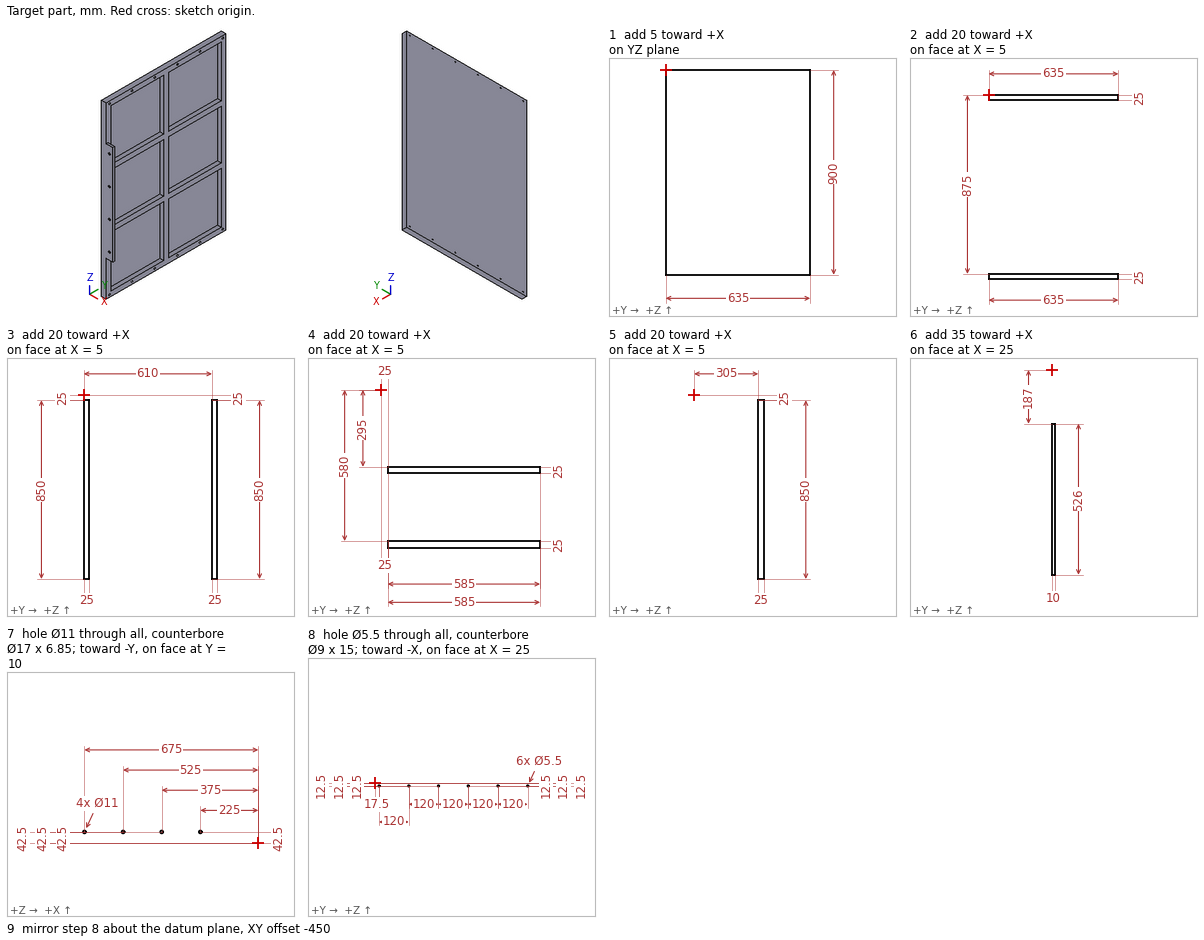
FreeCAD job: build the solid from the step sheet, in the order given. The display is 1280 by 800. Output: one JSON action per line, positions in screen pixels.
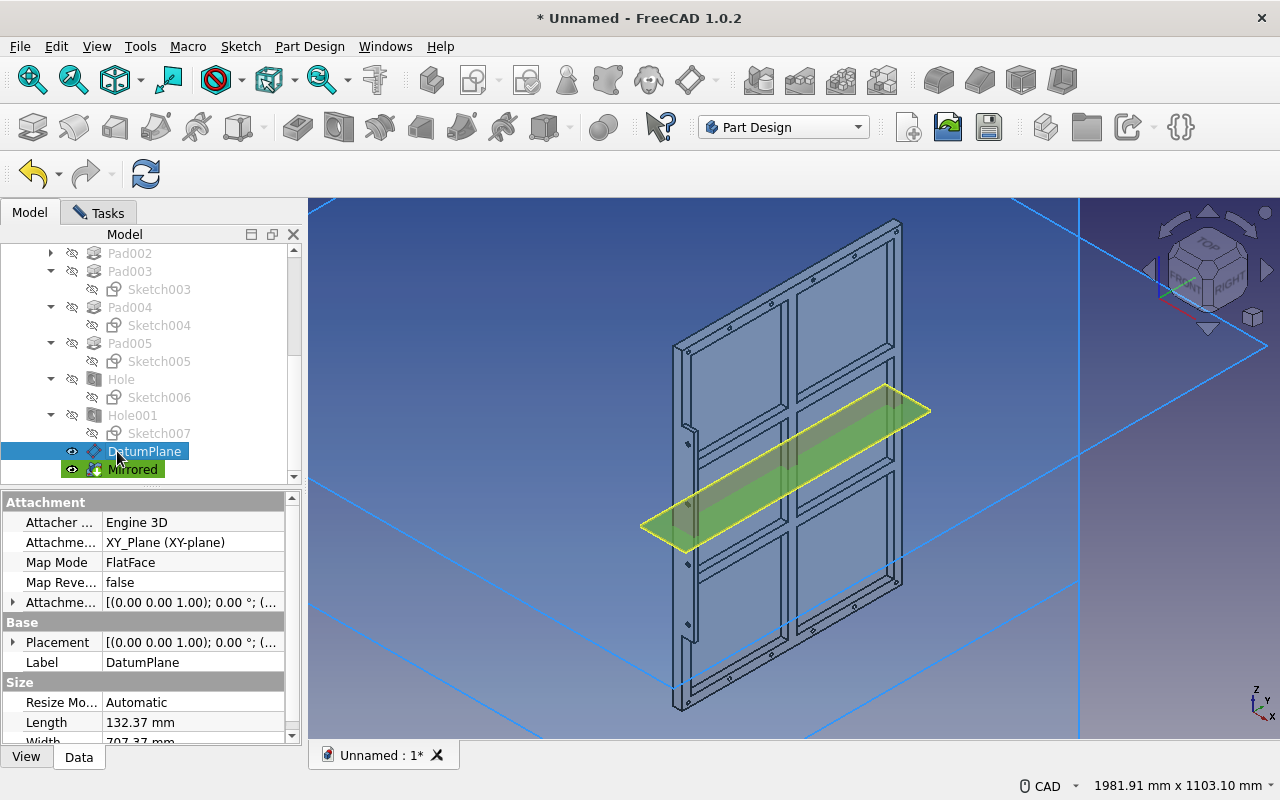
{"action": "left_click", "coordinate": [98, 212]}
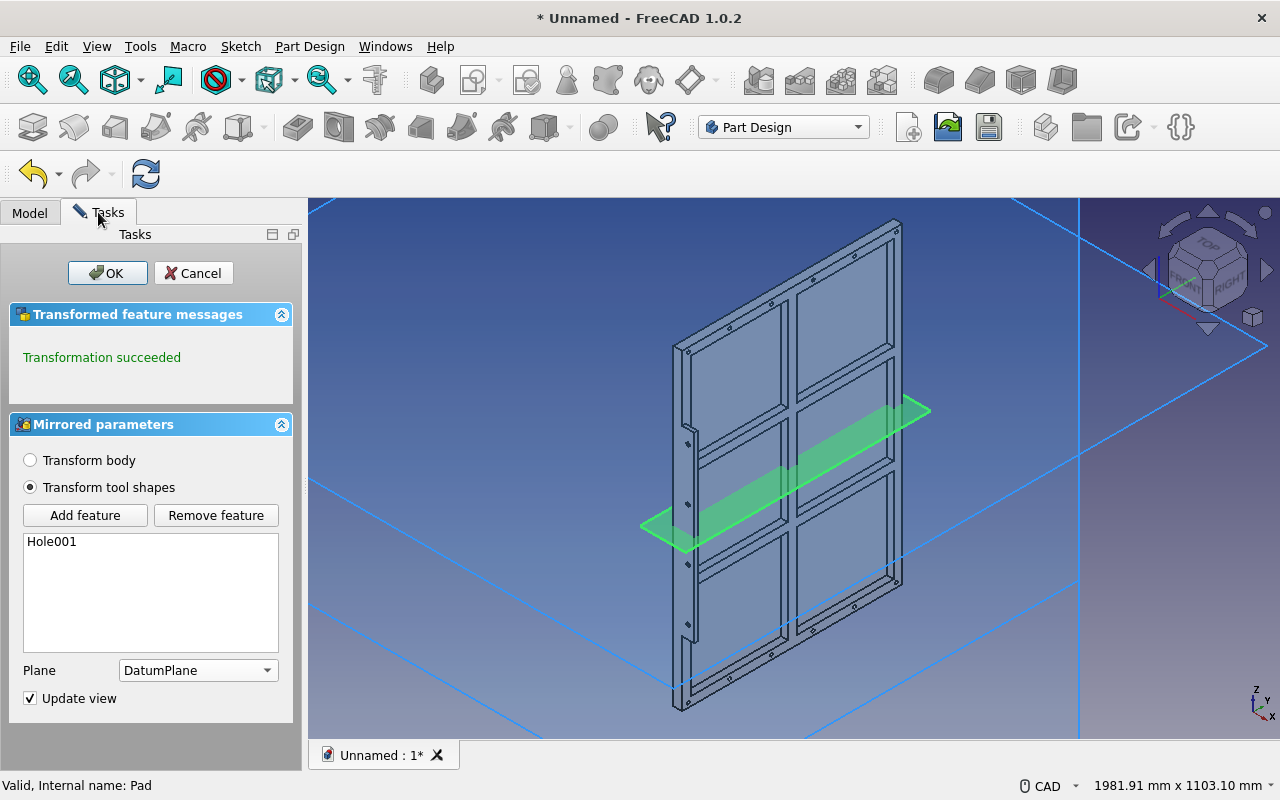
{"action": "left_click", "coordinate": [108, 273]}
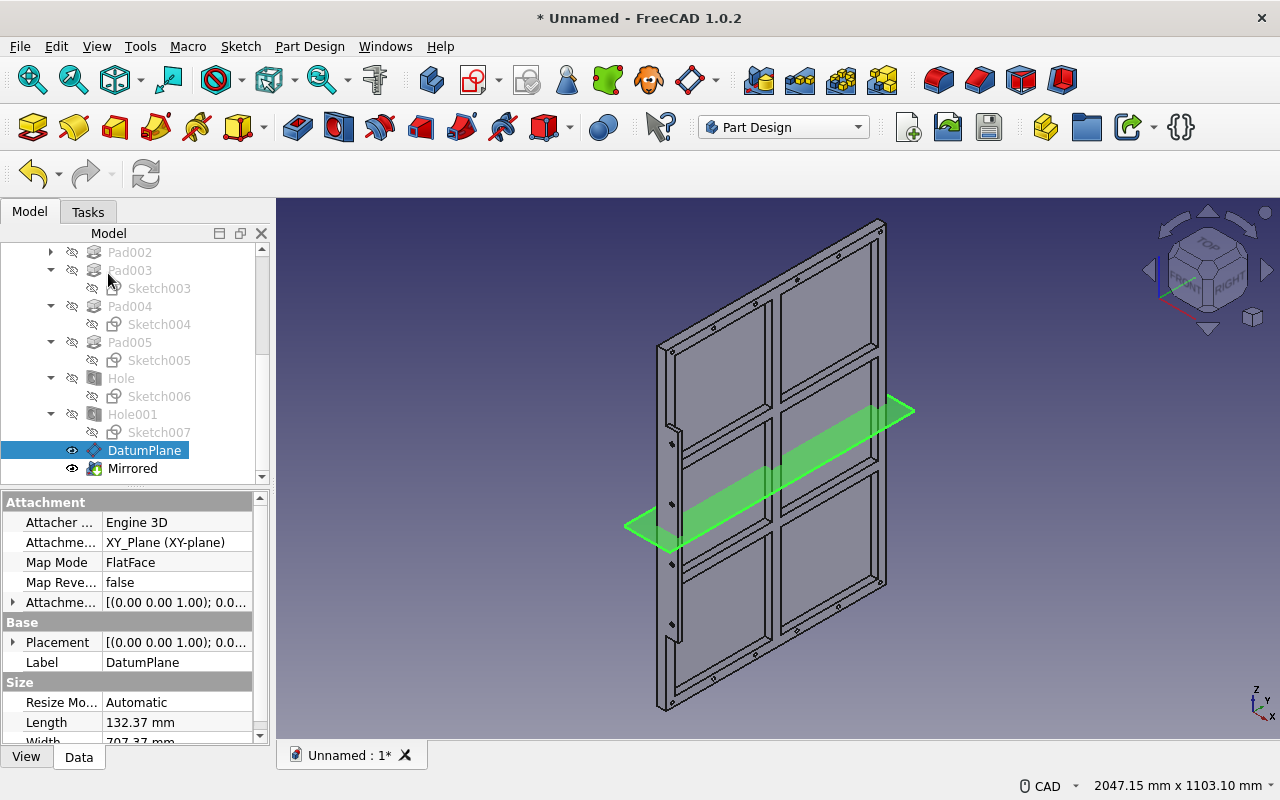
{"action": "left_click", "coordinate": [117, 450]}
{"action": "key", "text": "space"}